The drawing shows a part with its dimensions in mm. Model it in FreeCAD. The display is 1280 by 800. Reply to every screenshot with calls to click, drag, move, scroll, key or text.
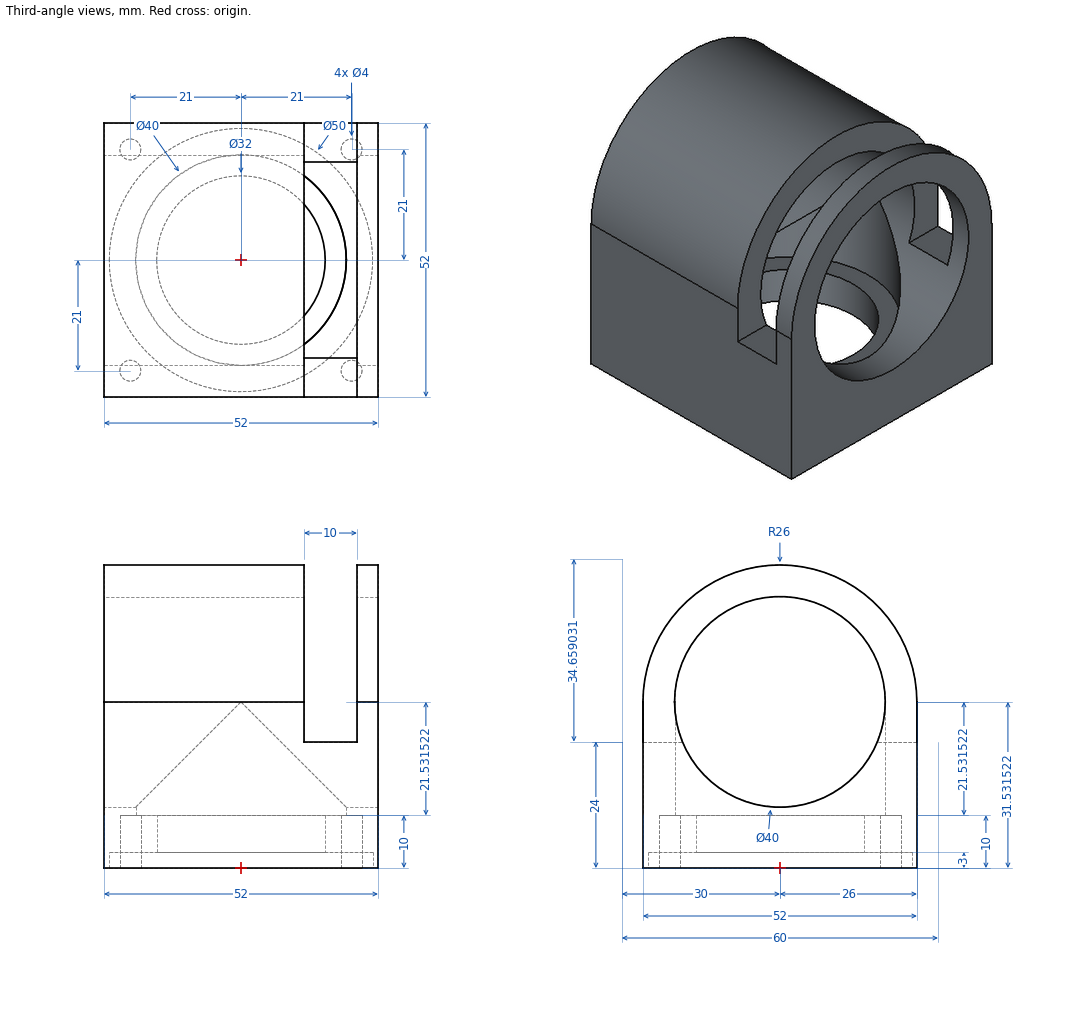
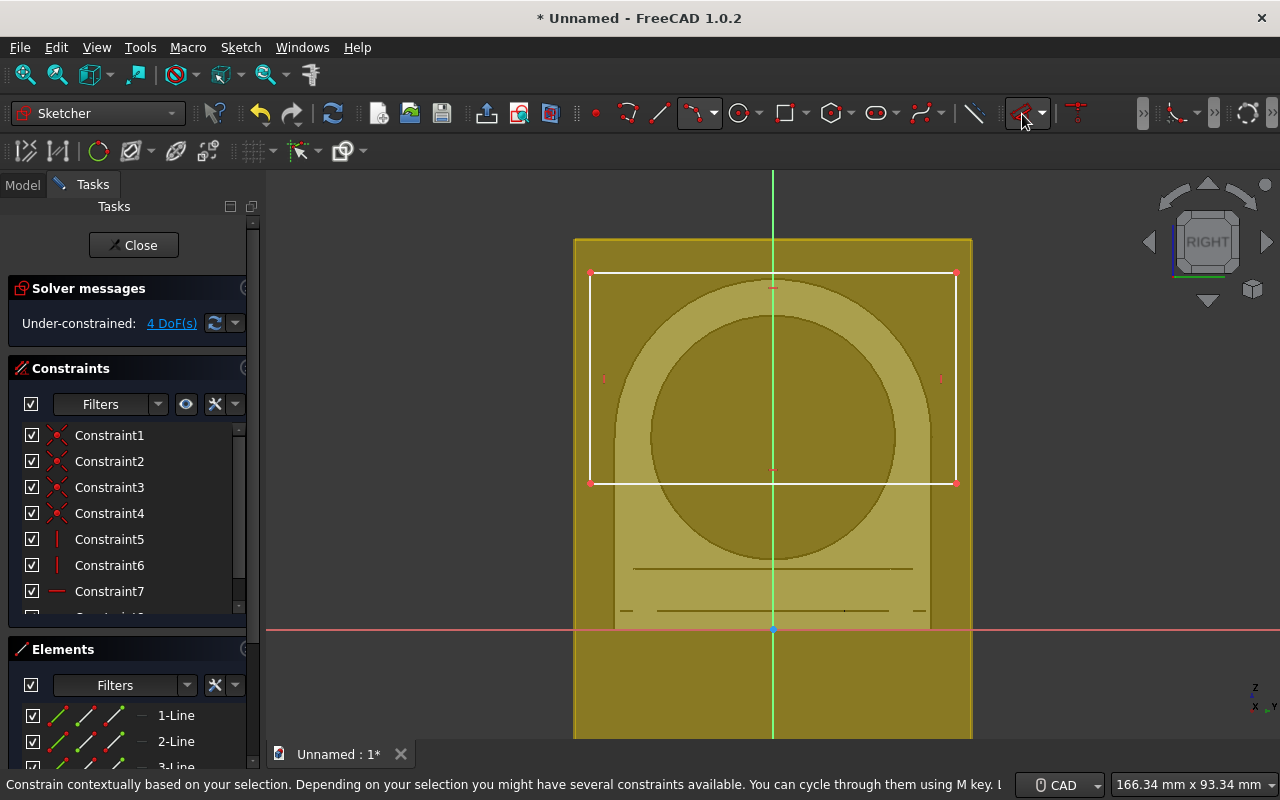
click(700, 484)
click(689, 518)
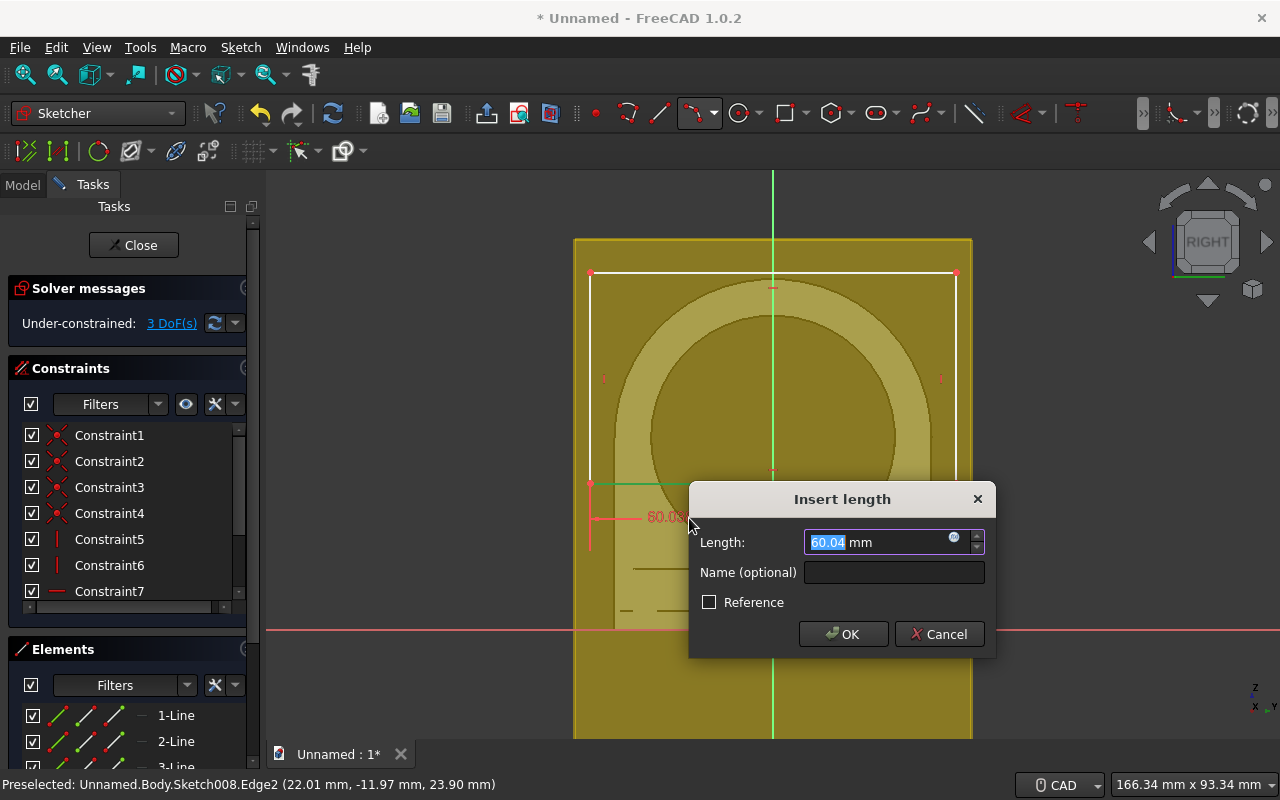
text(60)
key(Return)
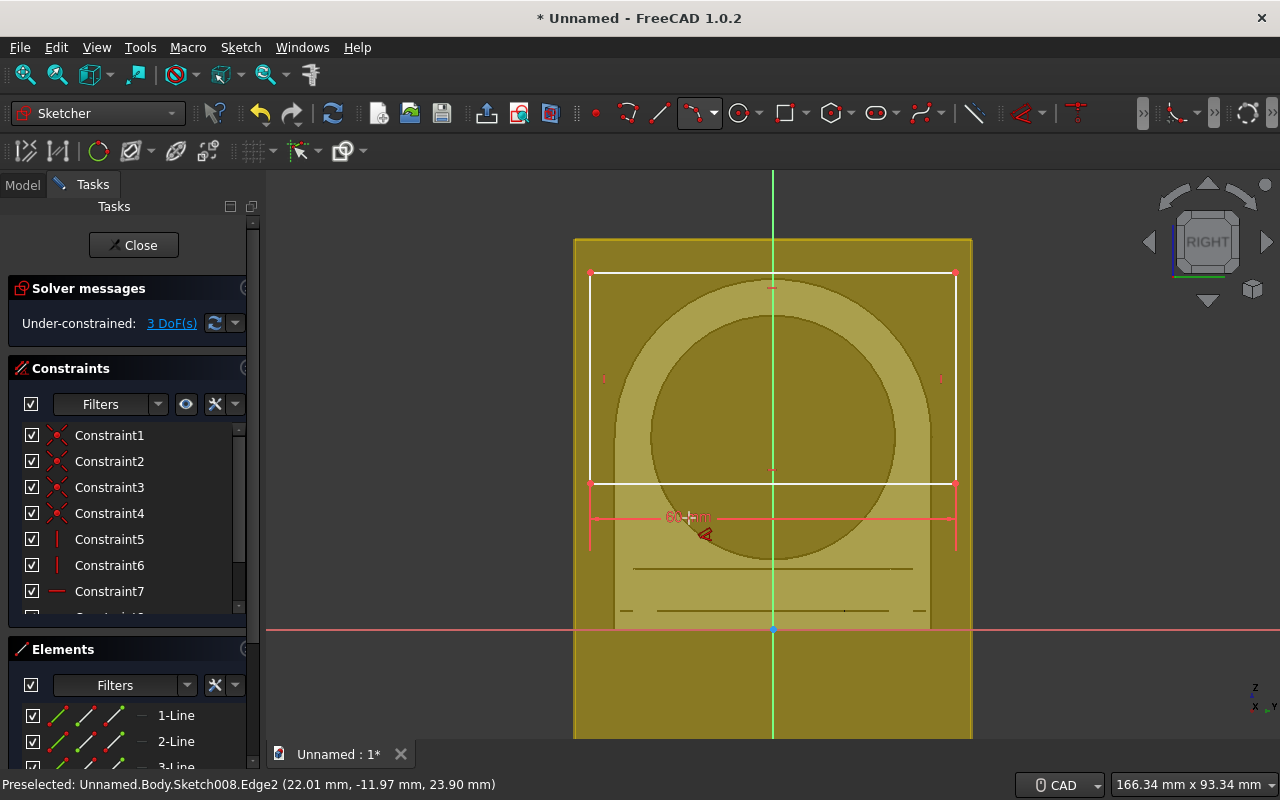
click(590, 273)
click(681, 664)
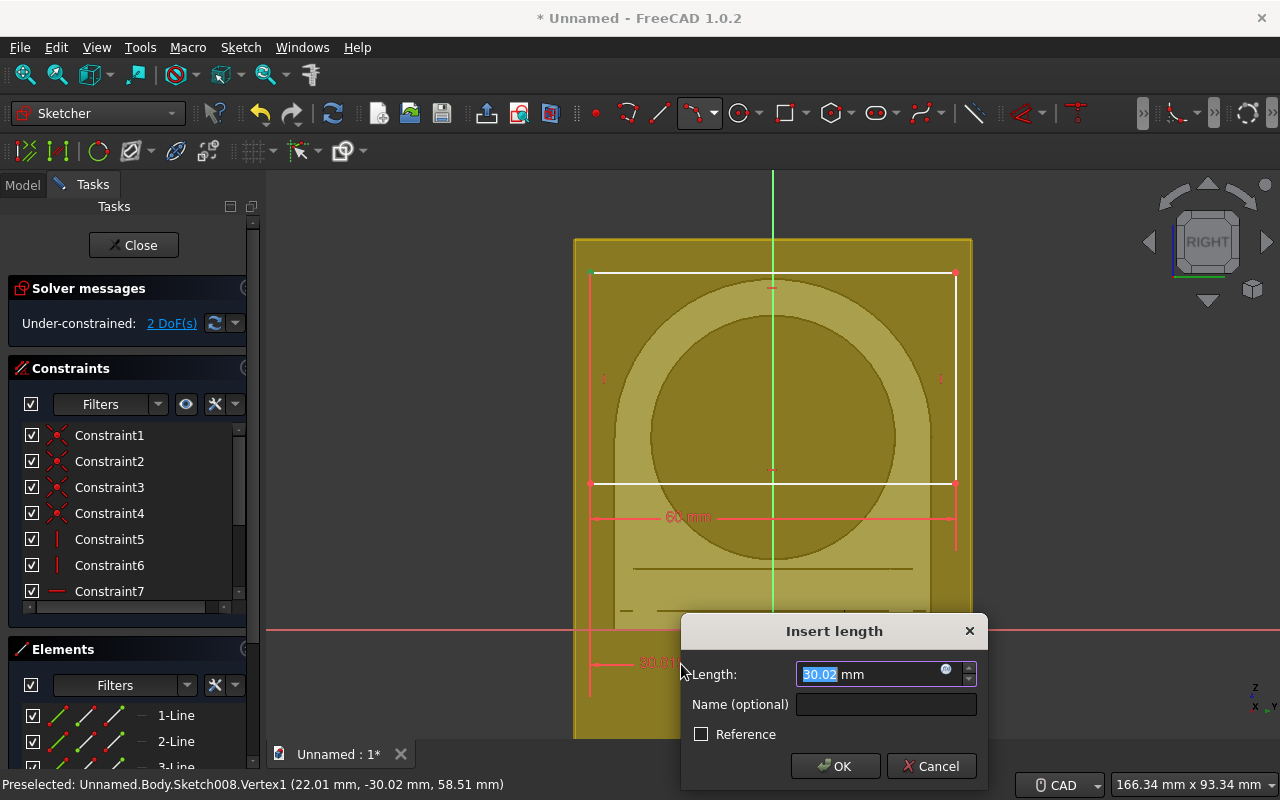
text(30)
key(Return)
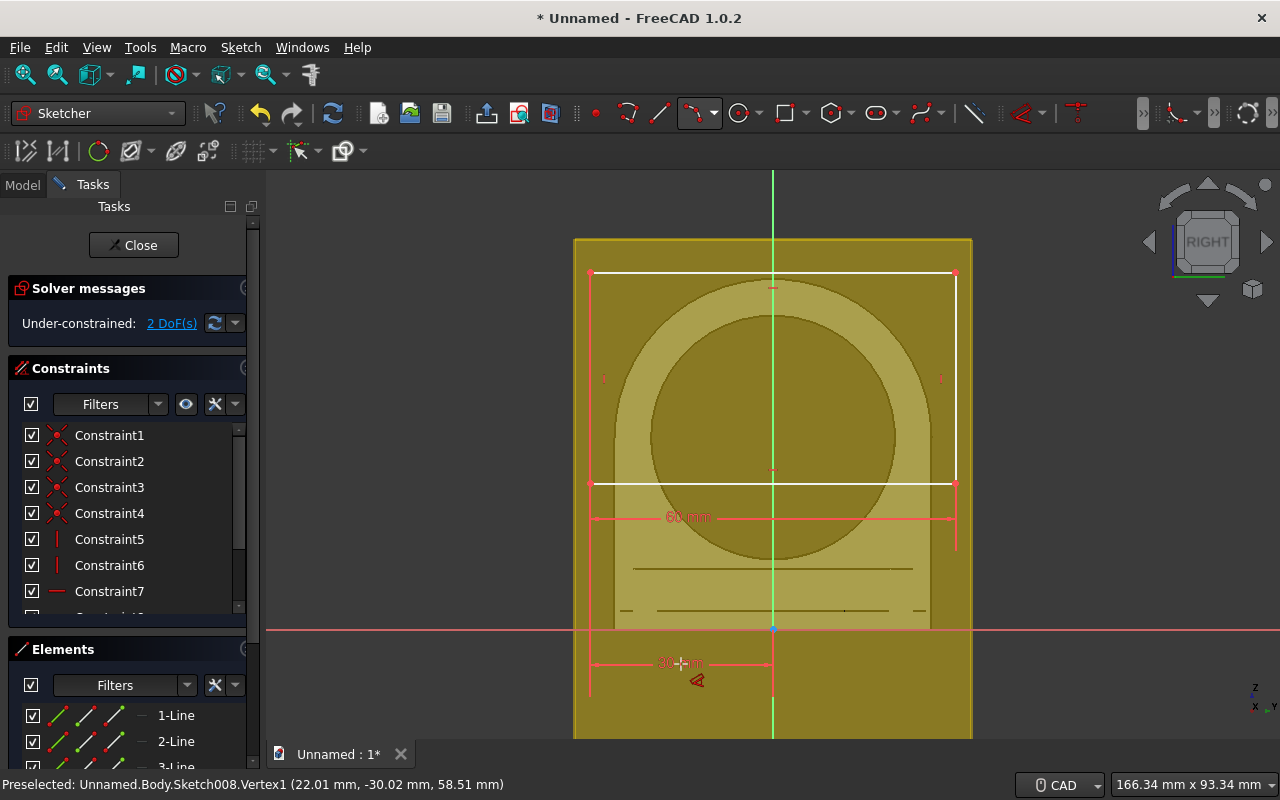
click(590, 484)
click(556, 557)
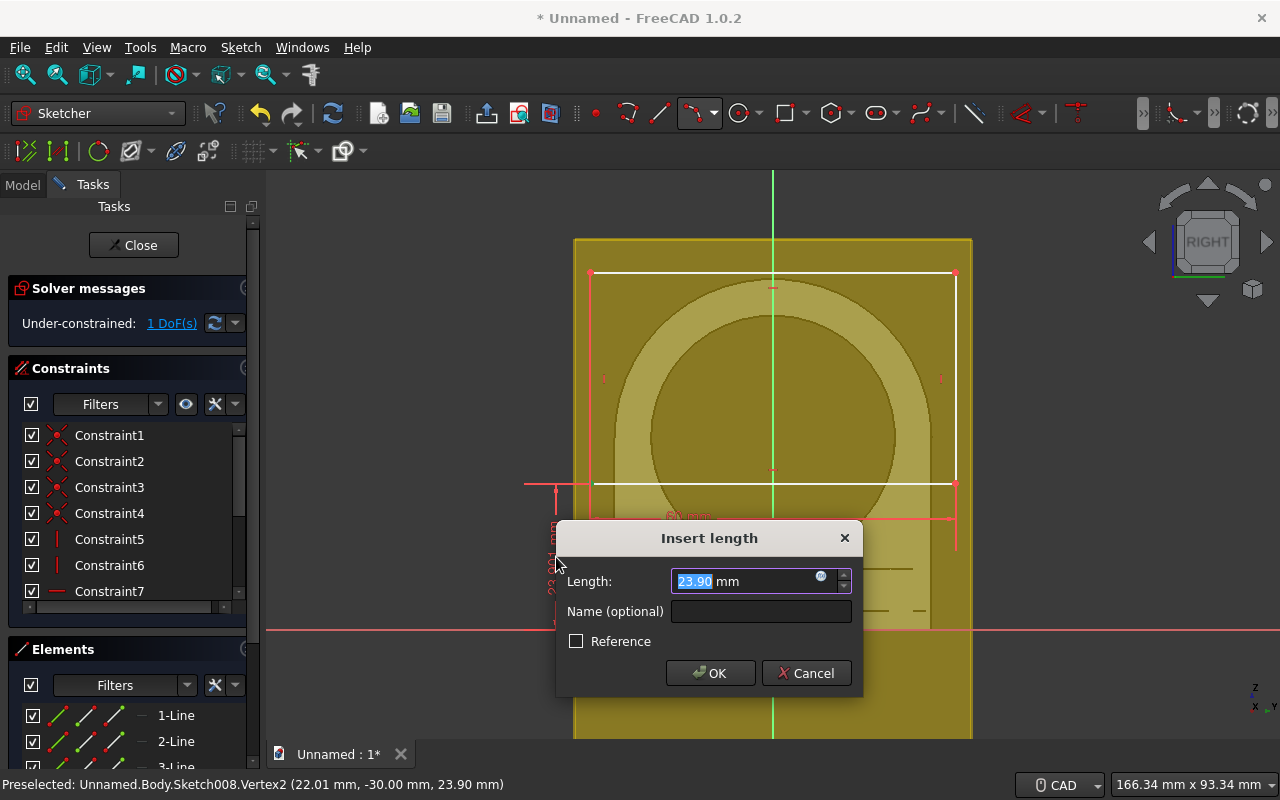
text(24)
key(Return)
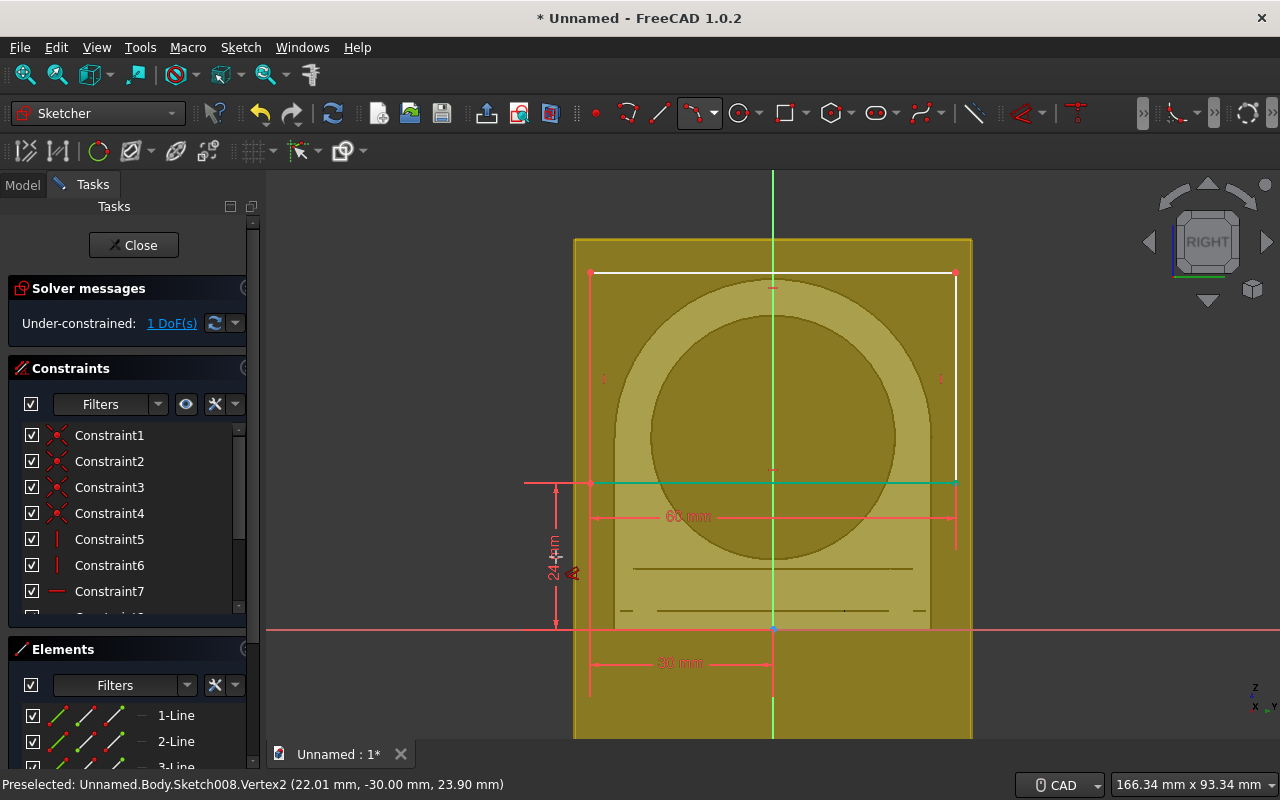
click(590, 336)
click(556, 378)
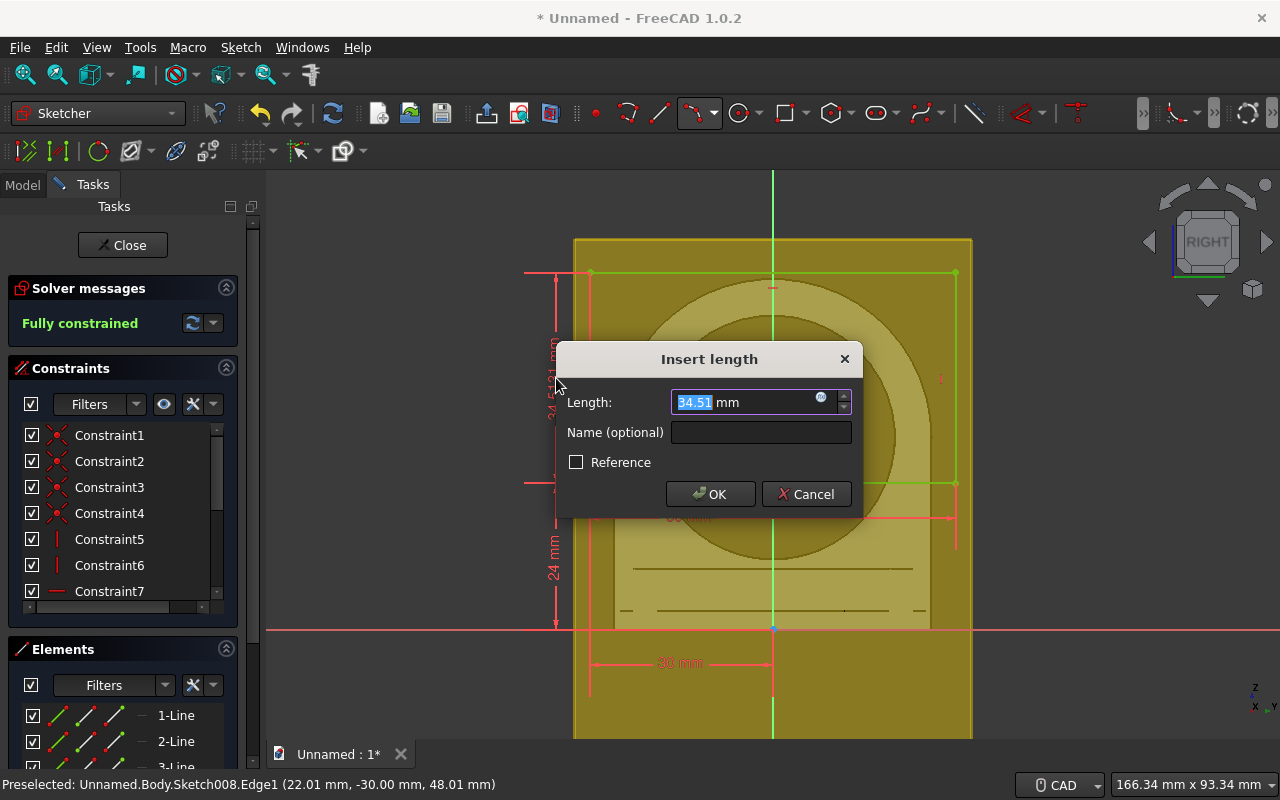
text(34.659031)
key(Return)
key(Escape)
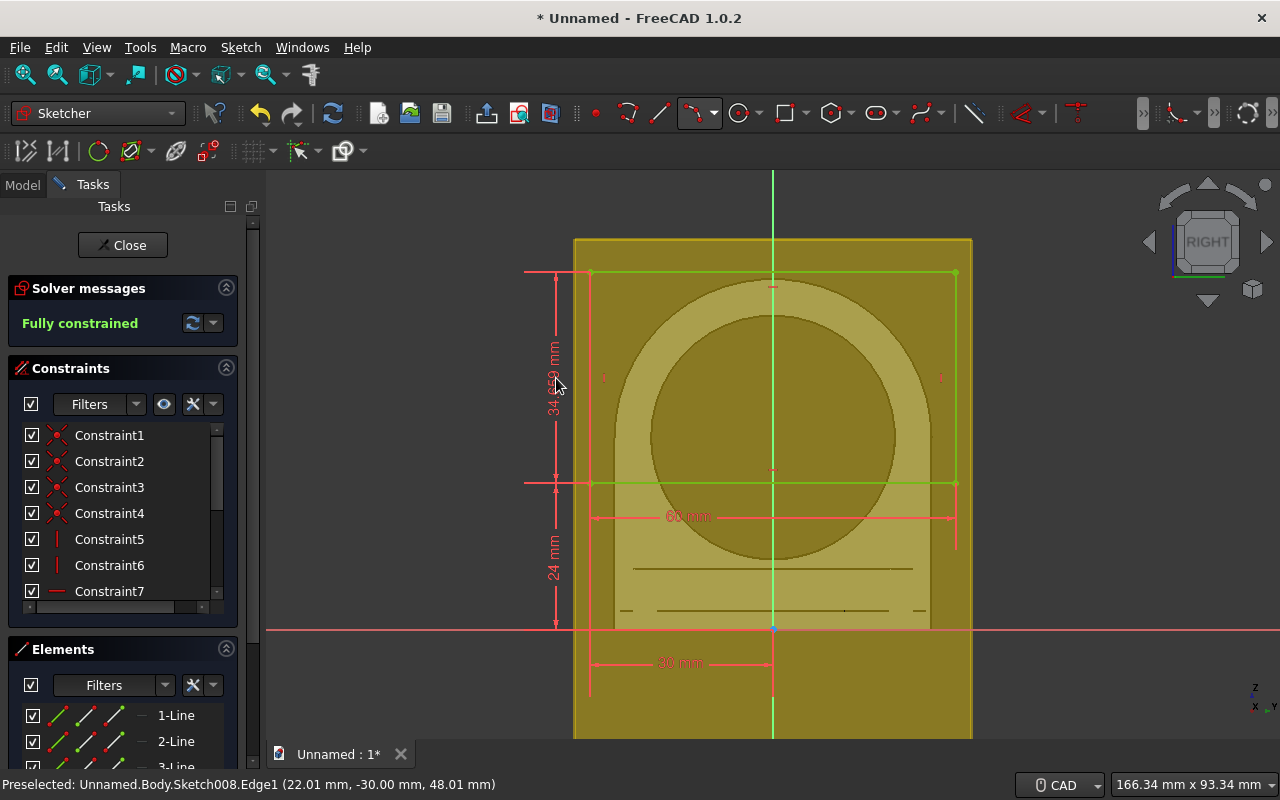
click(123, 245)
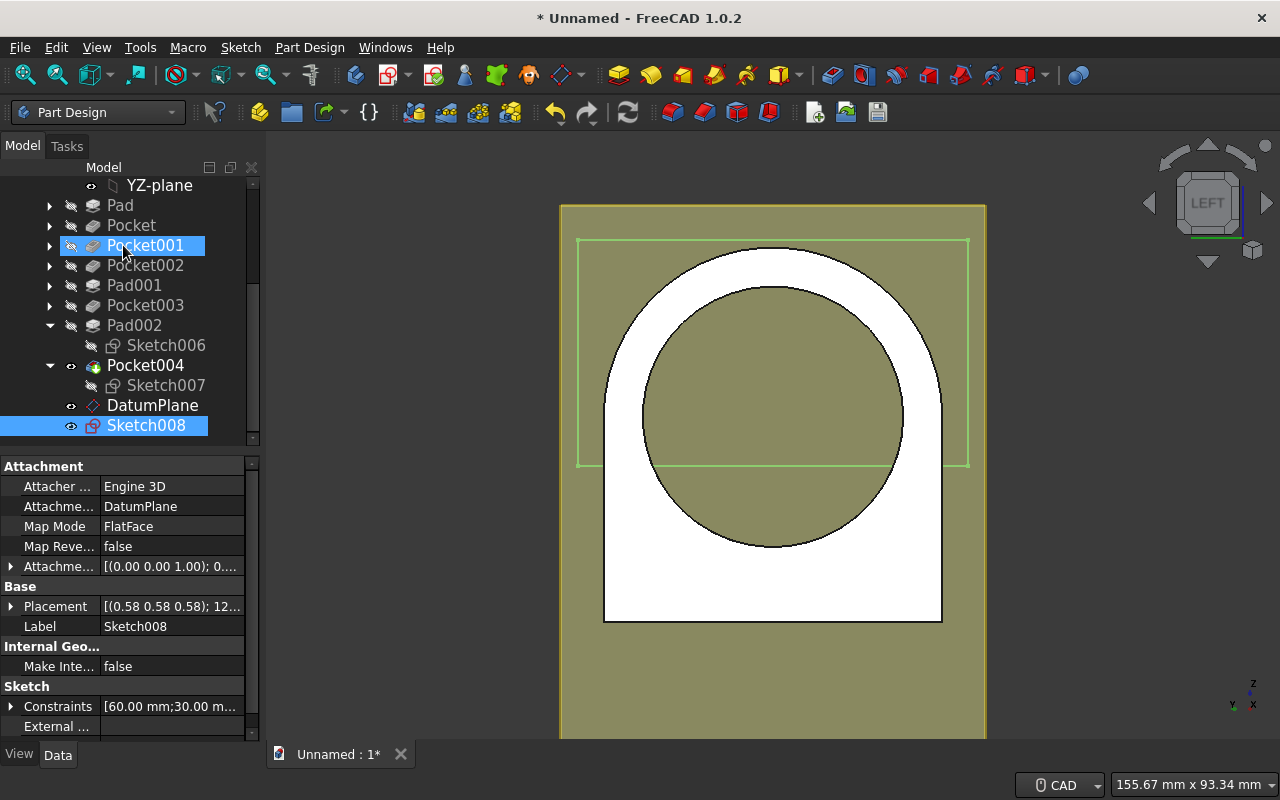
click(834, 76)